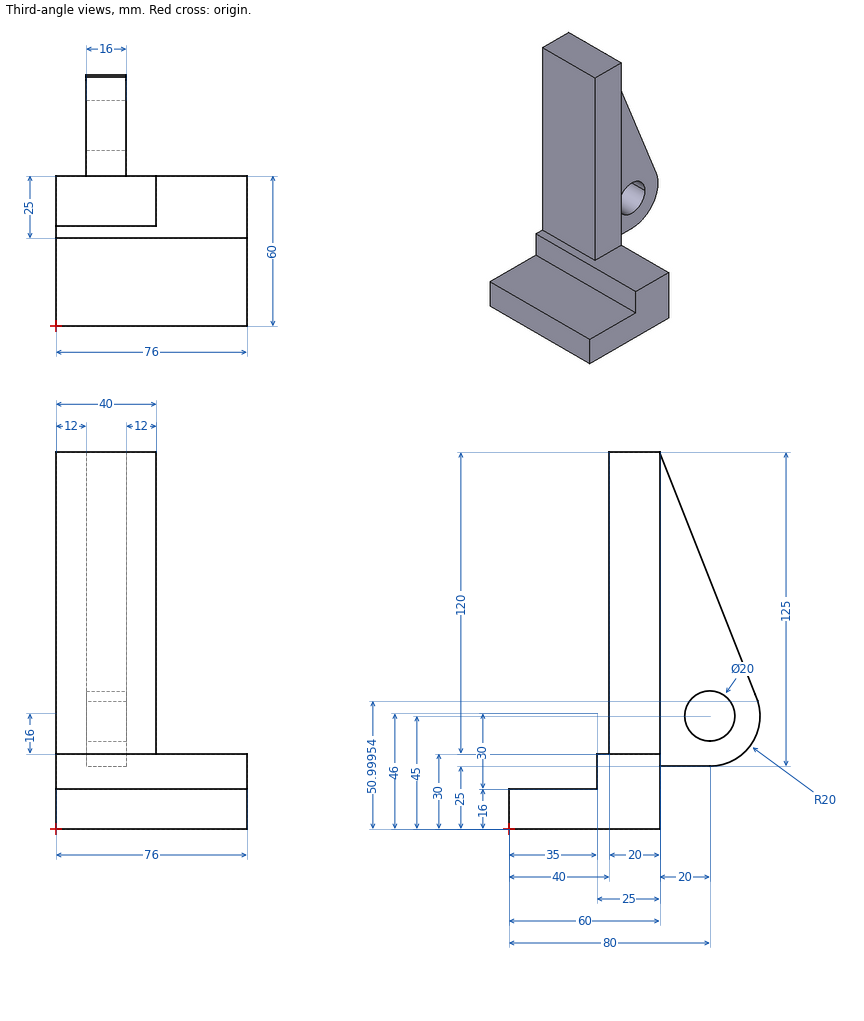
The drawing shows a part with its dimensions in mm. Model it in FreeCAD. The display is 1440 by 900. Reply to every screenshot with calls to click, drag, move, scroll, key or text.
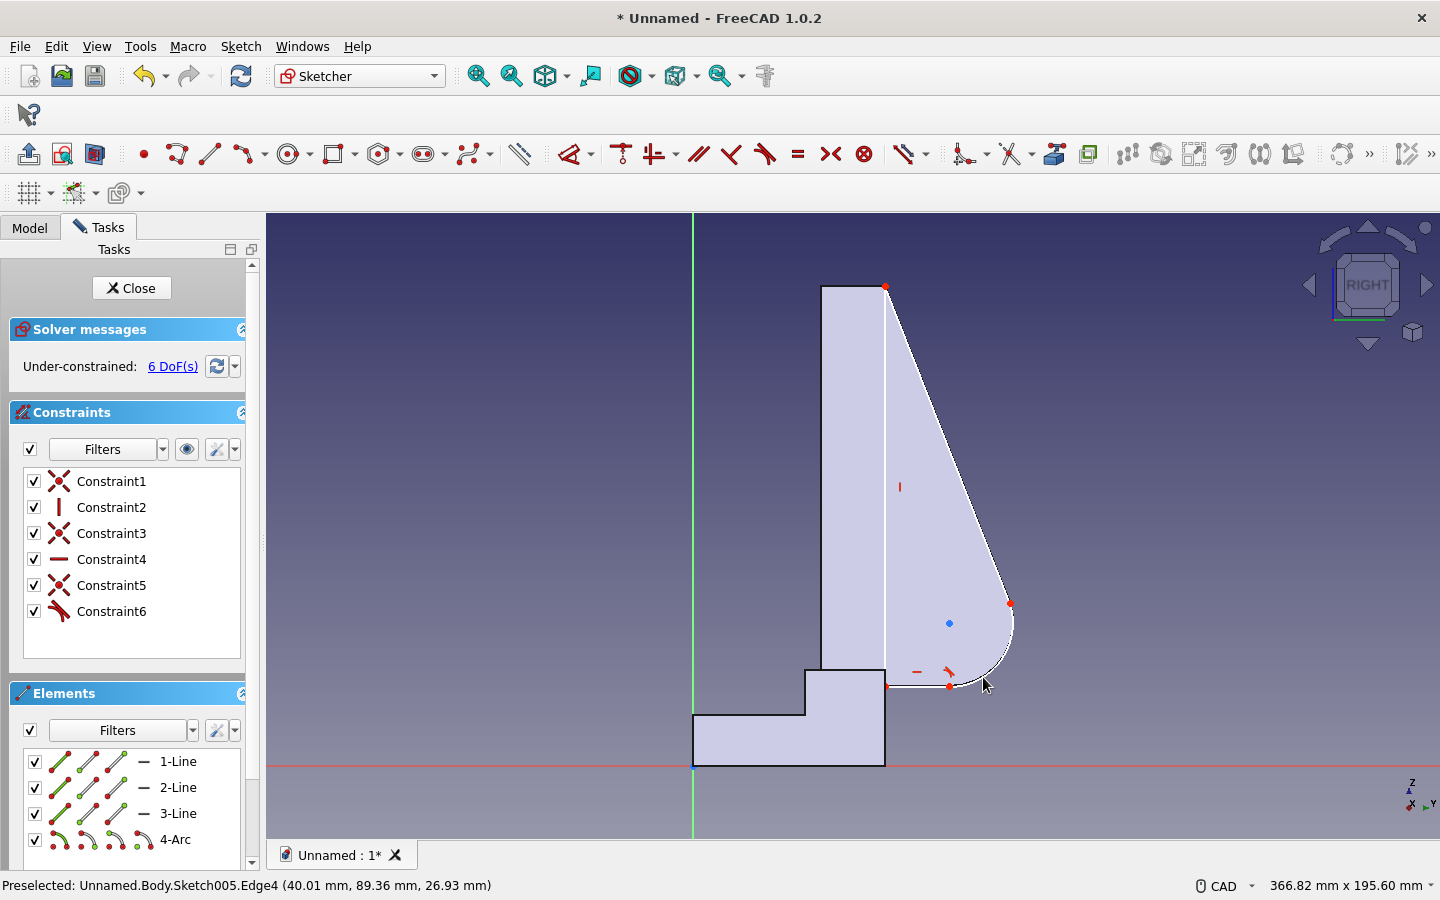
key(d)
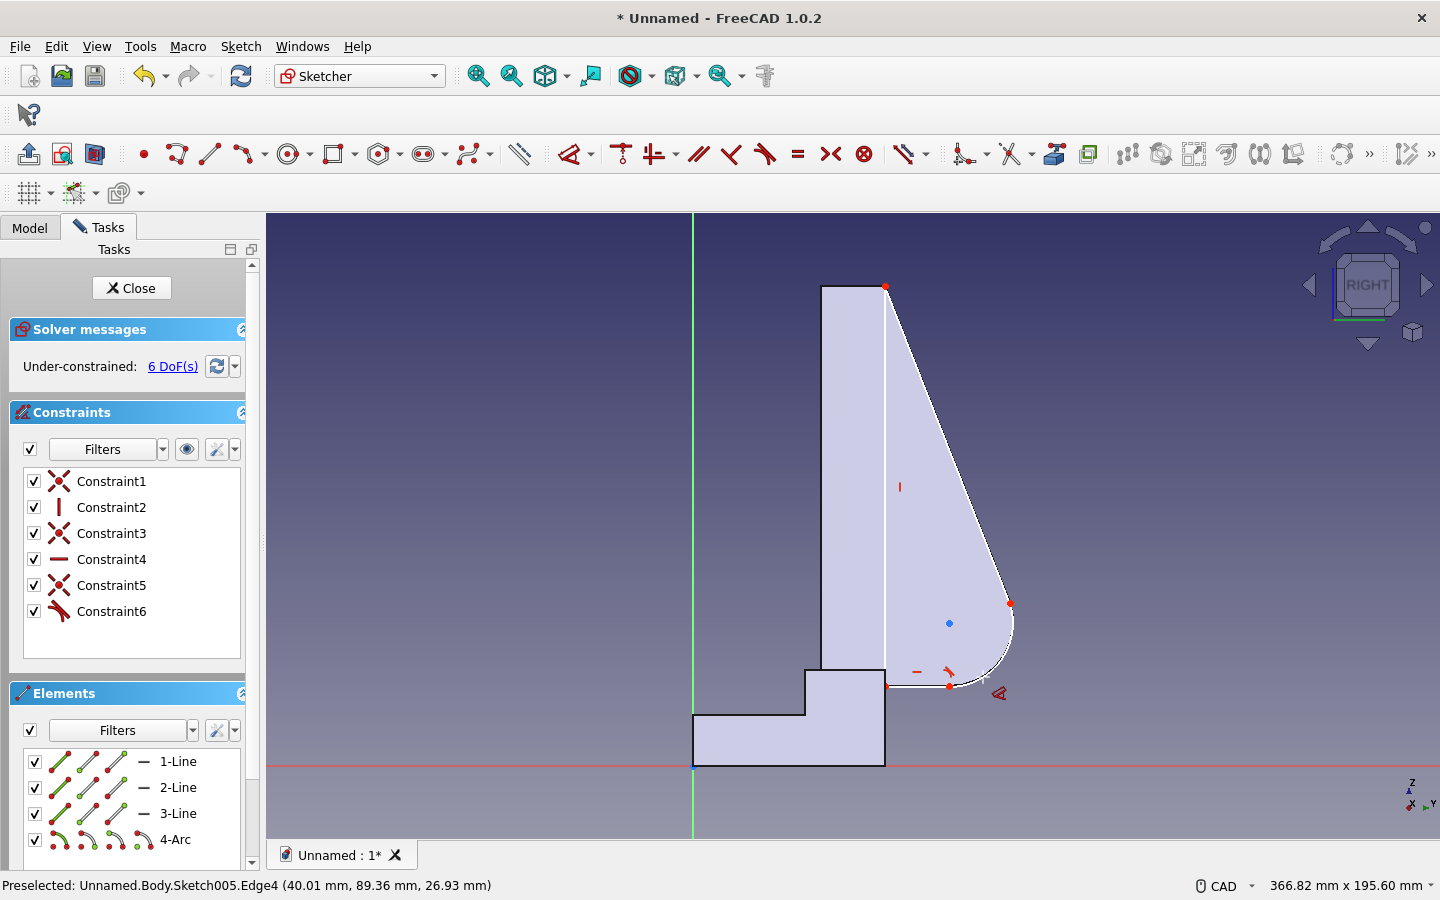
click(983, 677)
click(1000, 704)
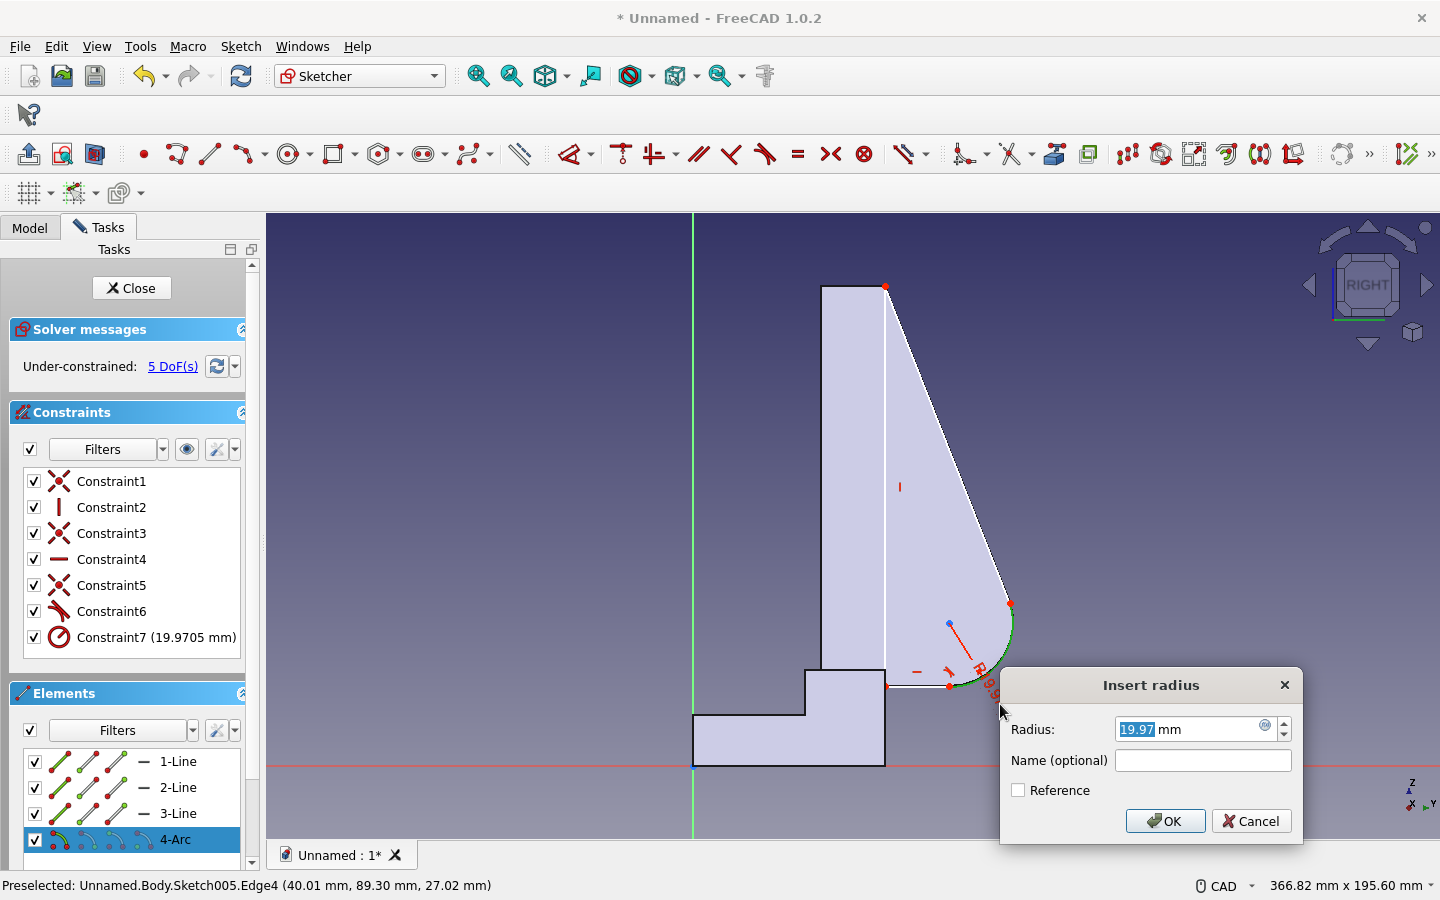
text(20)
key(Return)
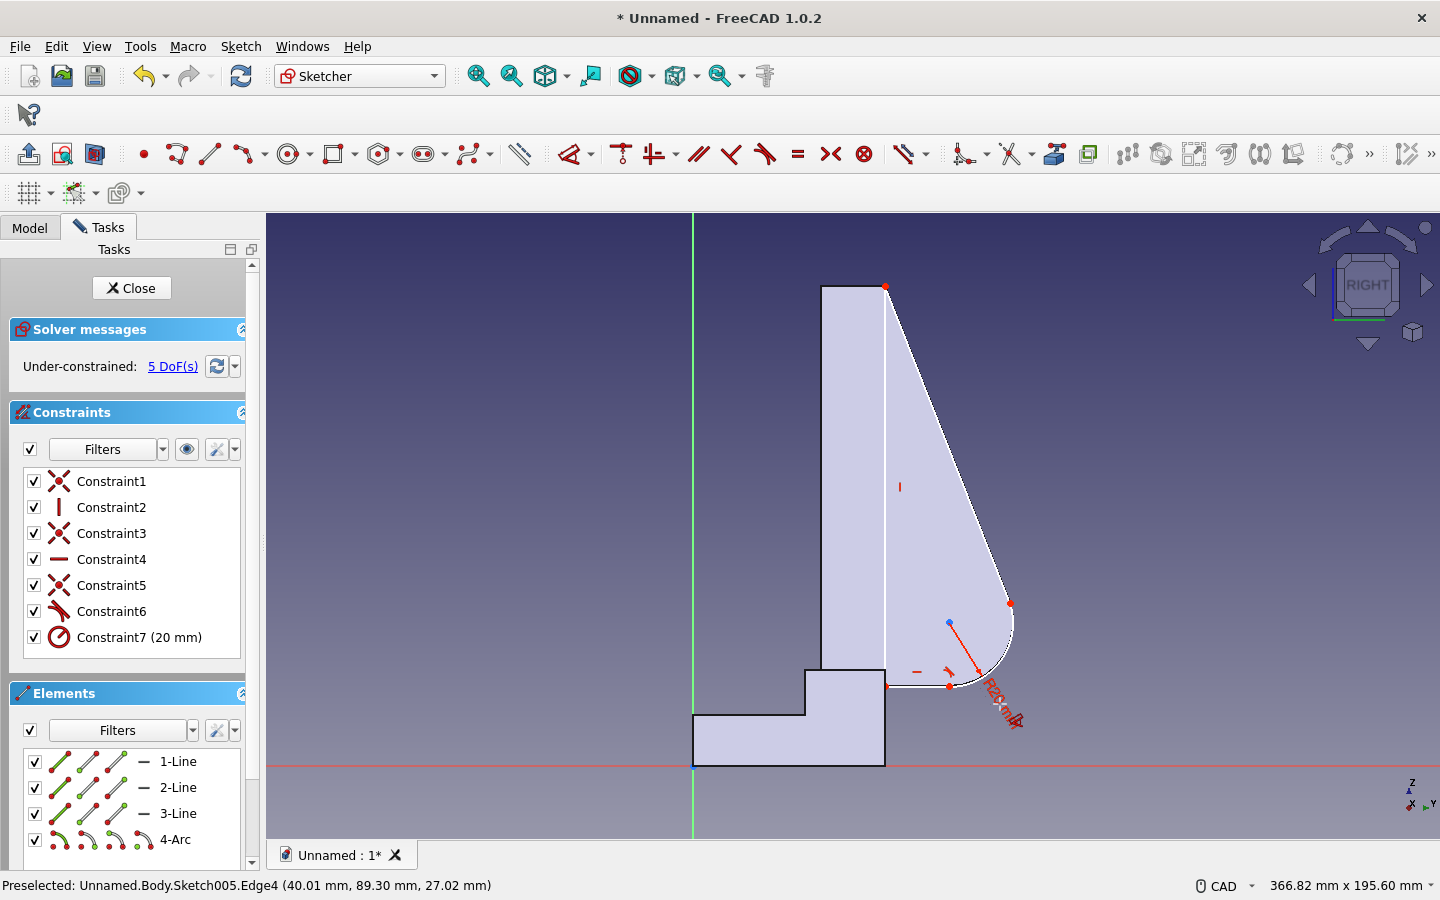
click(904, 687)
click(917, 721)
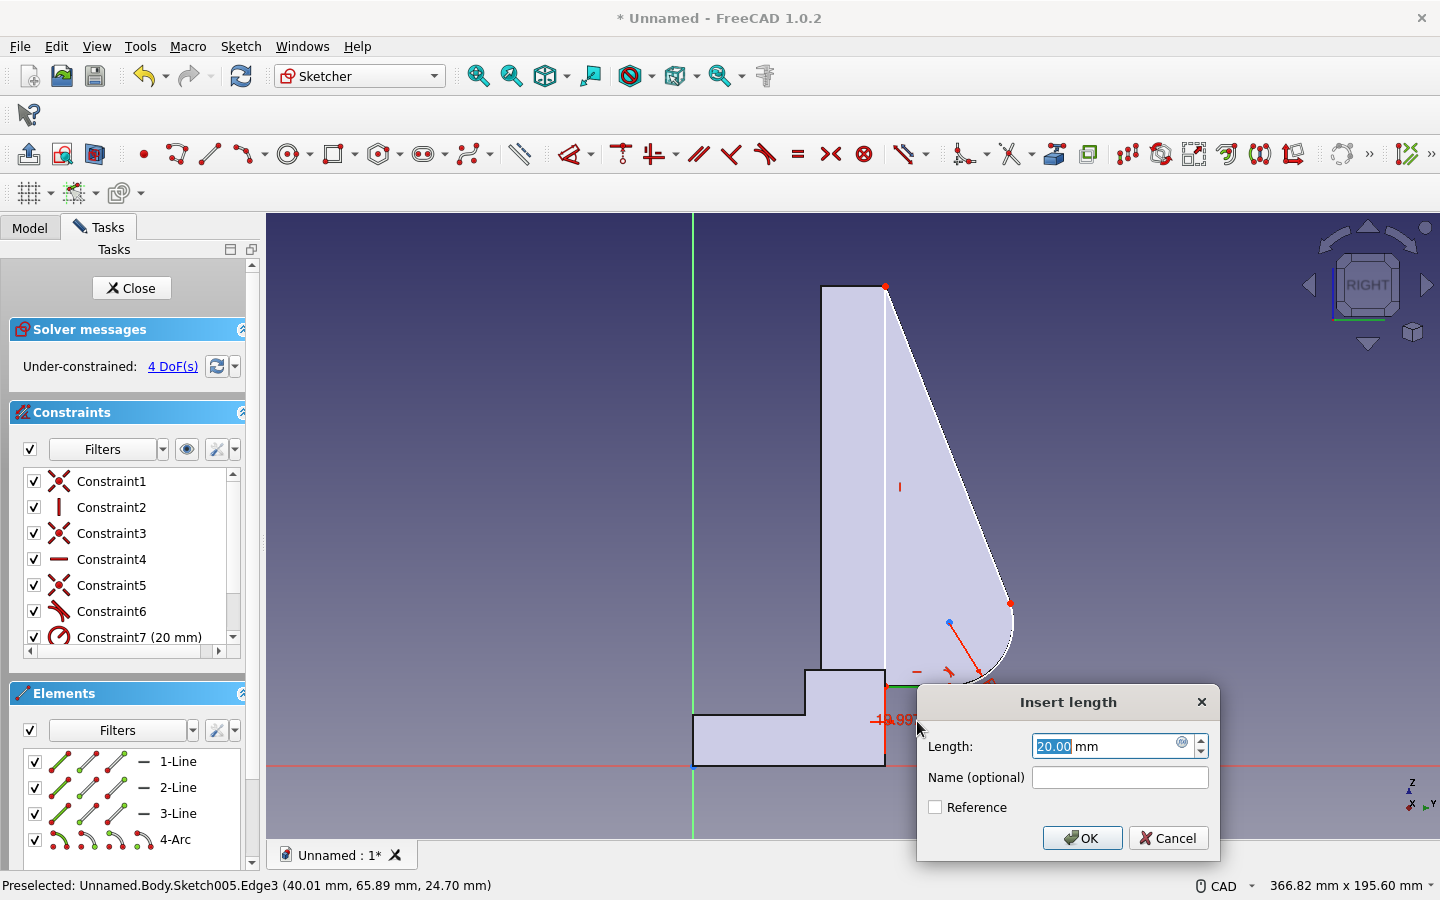
text(20)
key(Return)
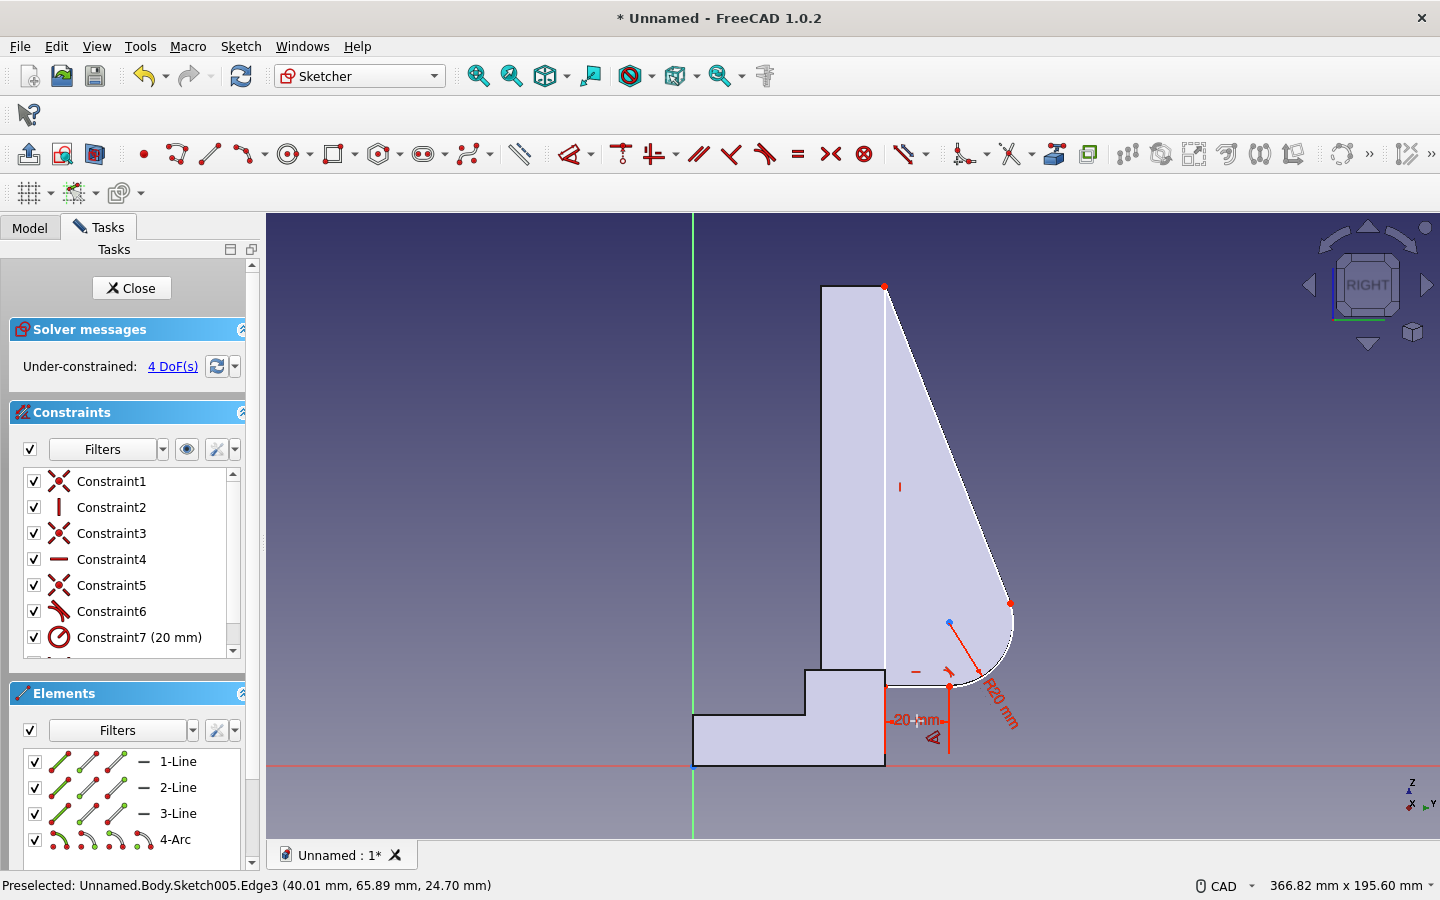
click(885, 407)
click(919, 487)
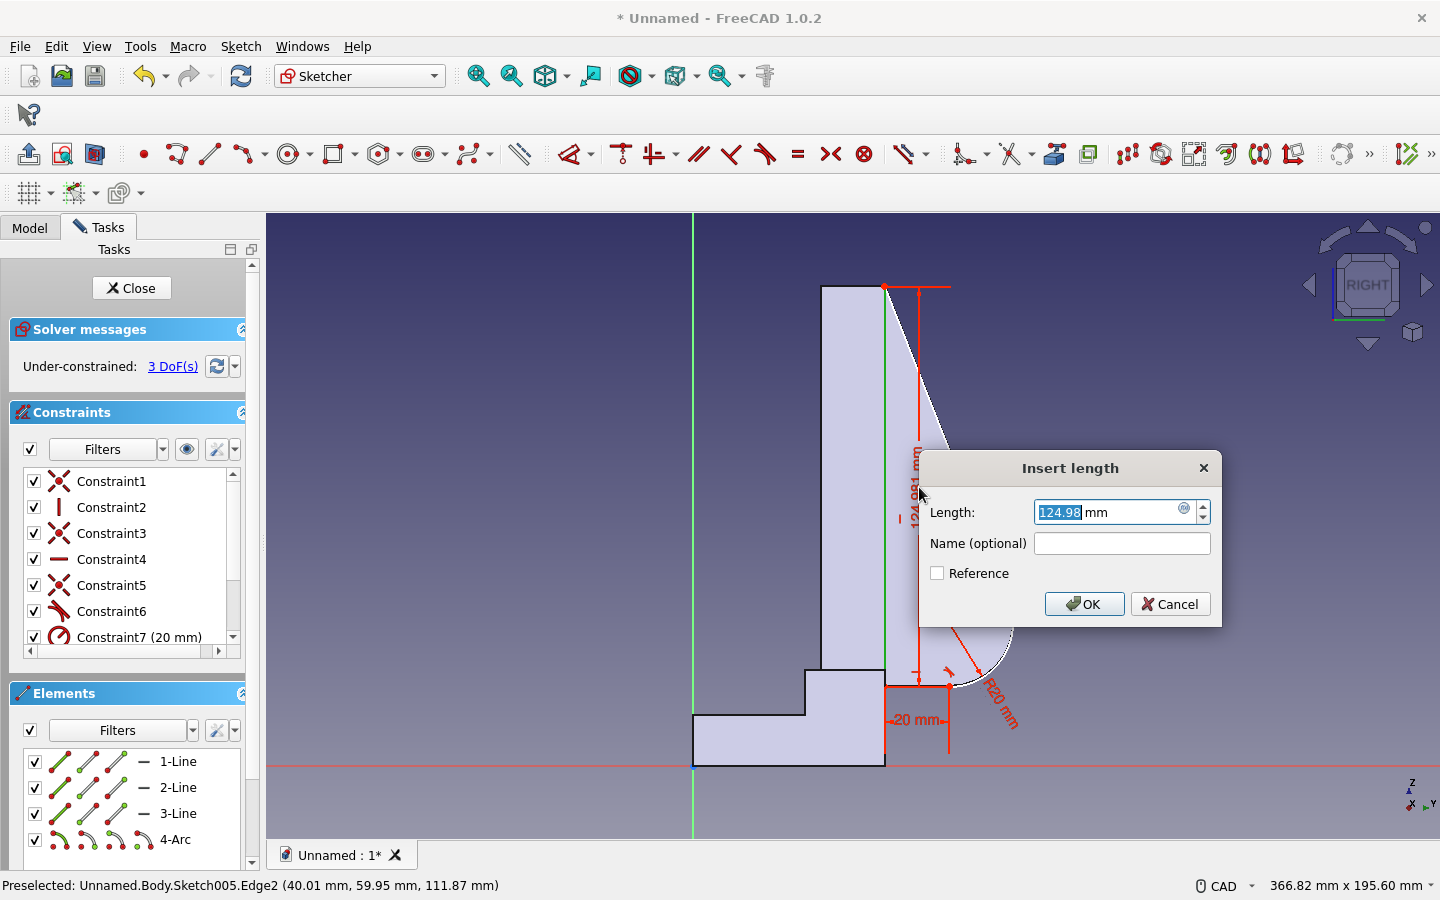
text(125)
key(Return)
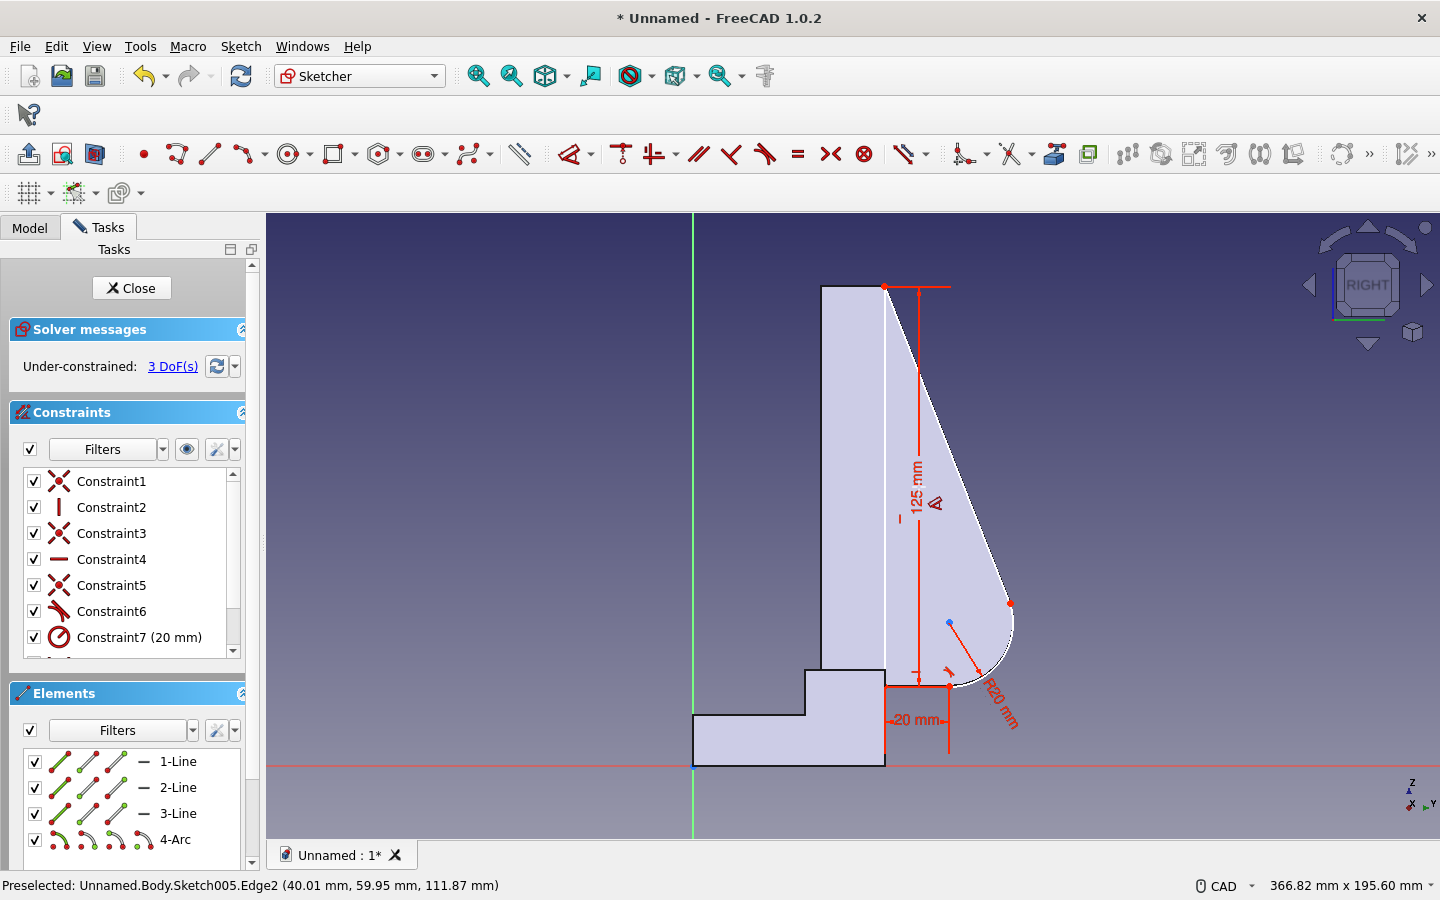
click(885, 287)
click(789, 800)